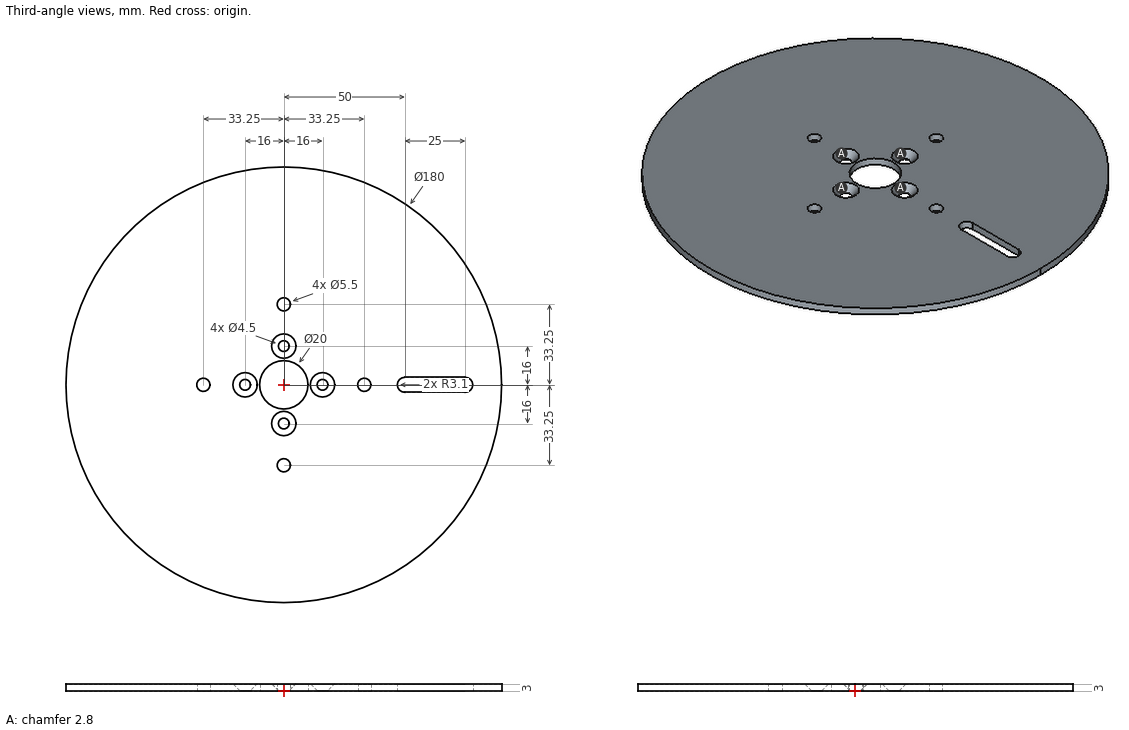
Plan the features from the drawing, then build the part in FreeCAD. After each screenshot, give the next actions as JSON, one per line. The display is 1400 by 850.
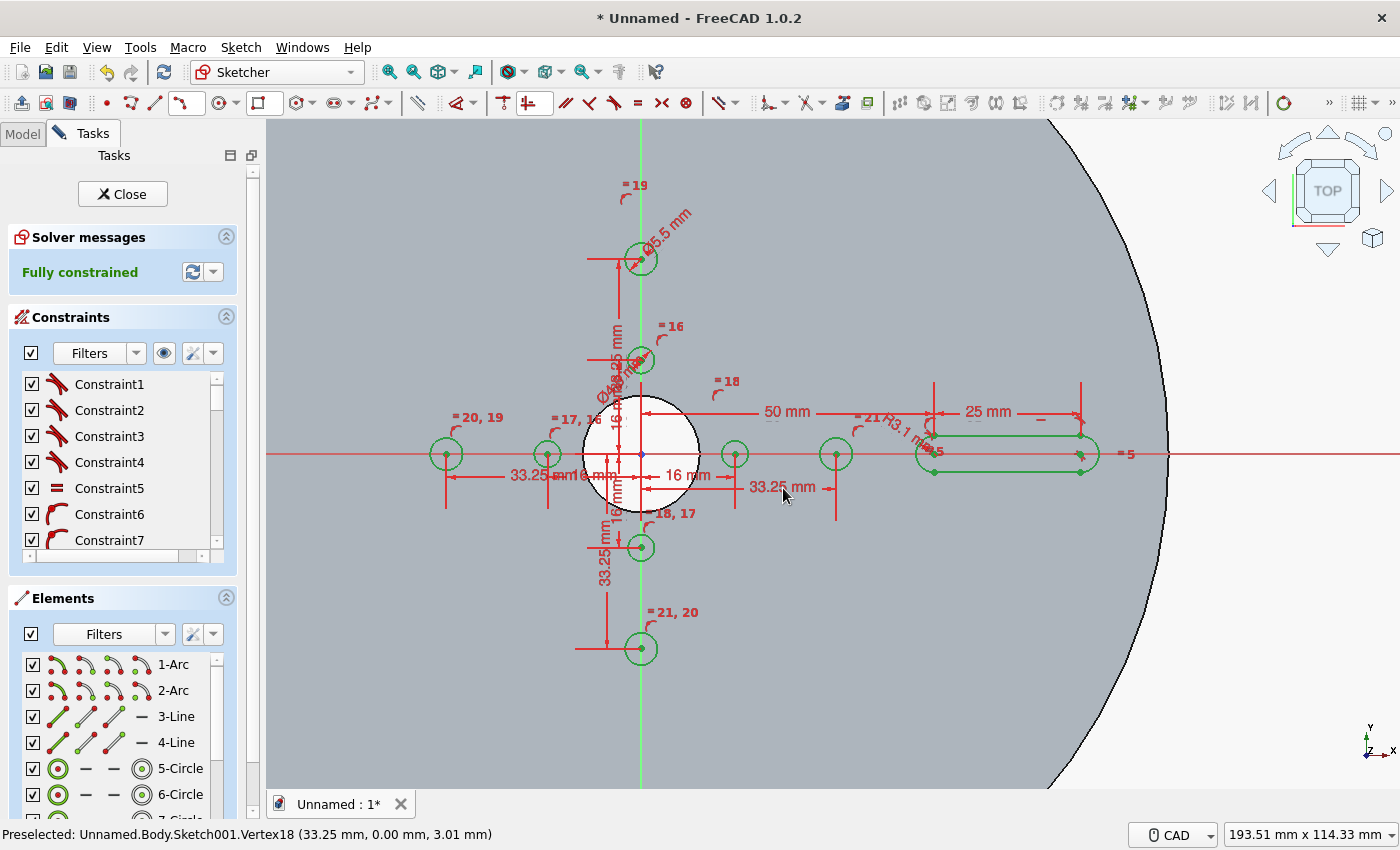
{"action": "left_click", "coordinate": [123, 194]}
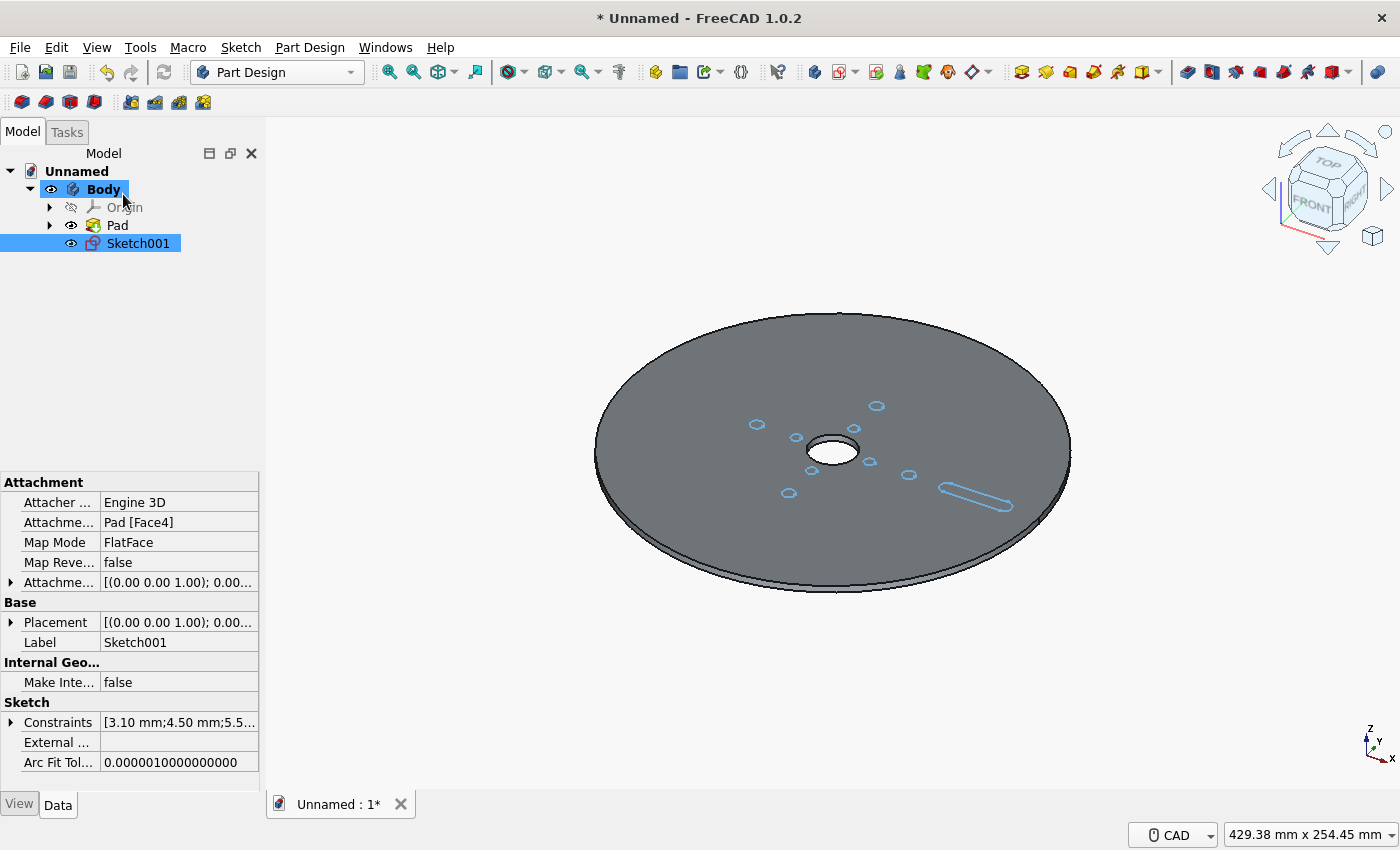
{"action": "left_click", "coordinate": [1188, 72]}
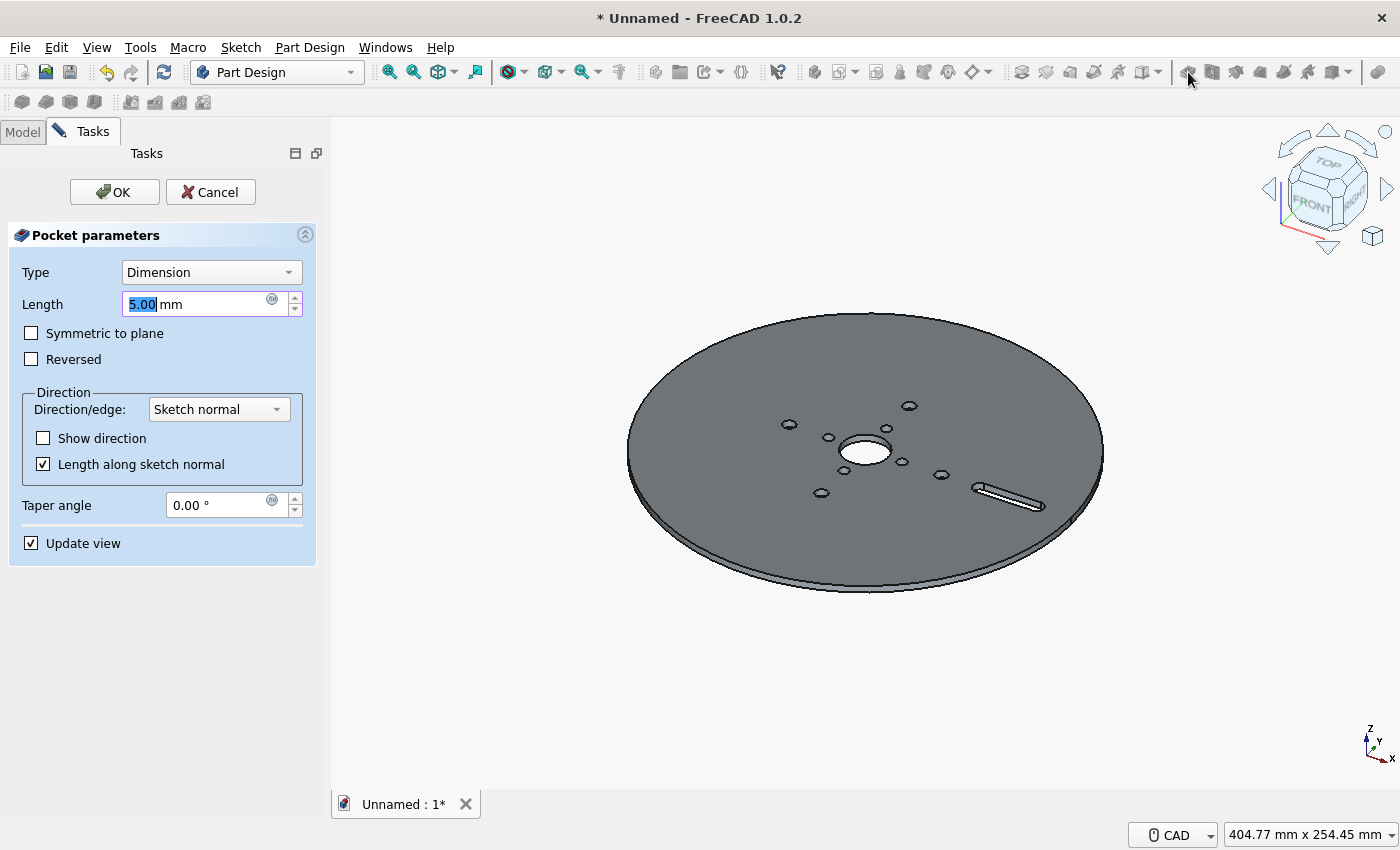
{"action": "type", "text": "3"}
{"action": "key", "text": "Tab"}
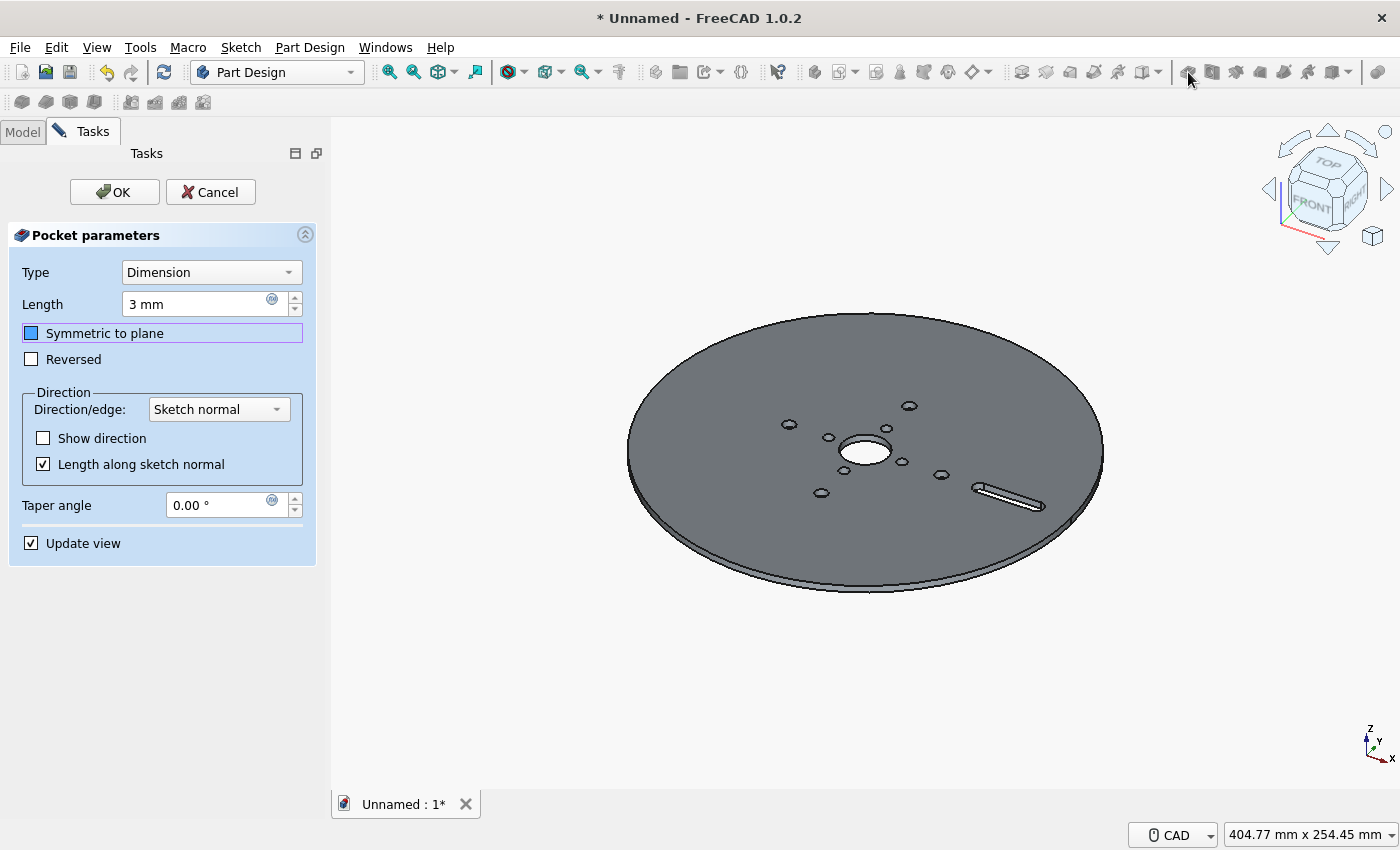
{"action": "left_click", "coordinate": [115, 192]}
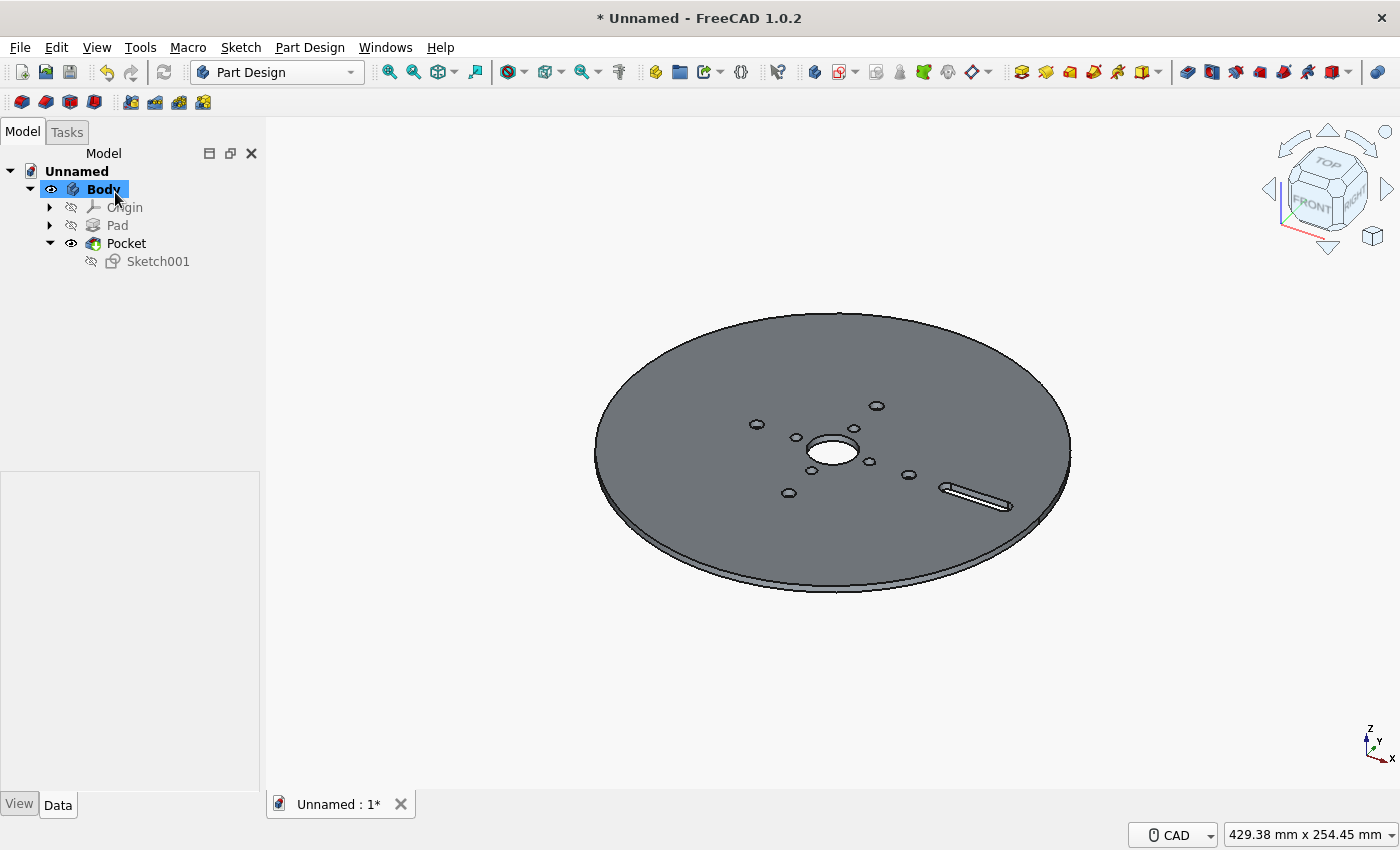
{"action": "left_click", "coordinate": [849, 426]}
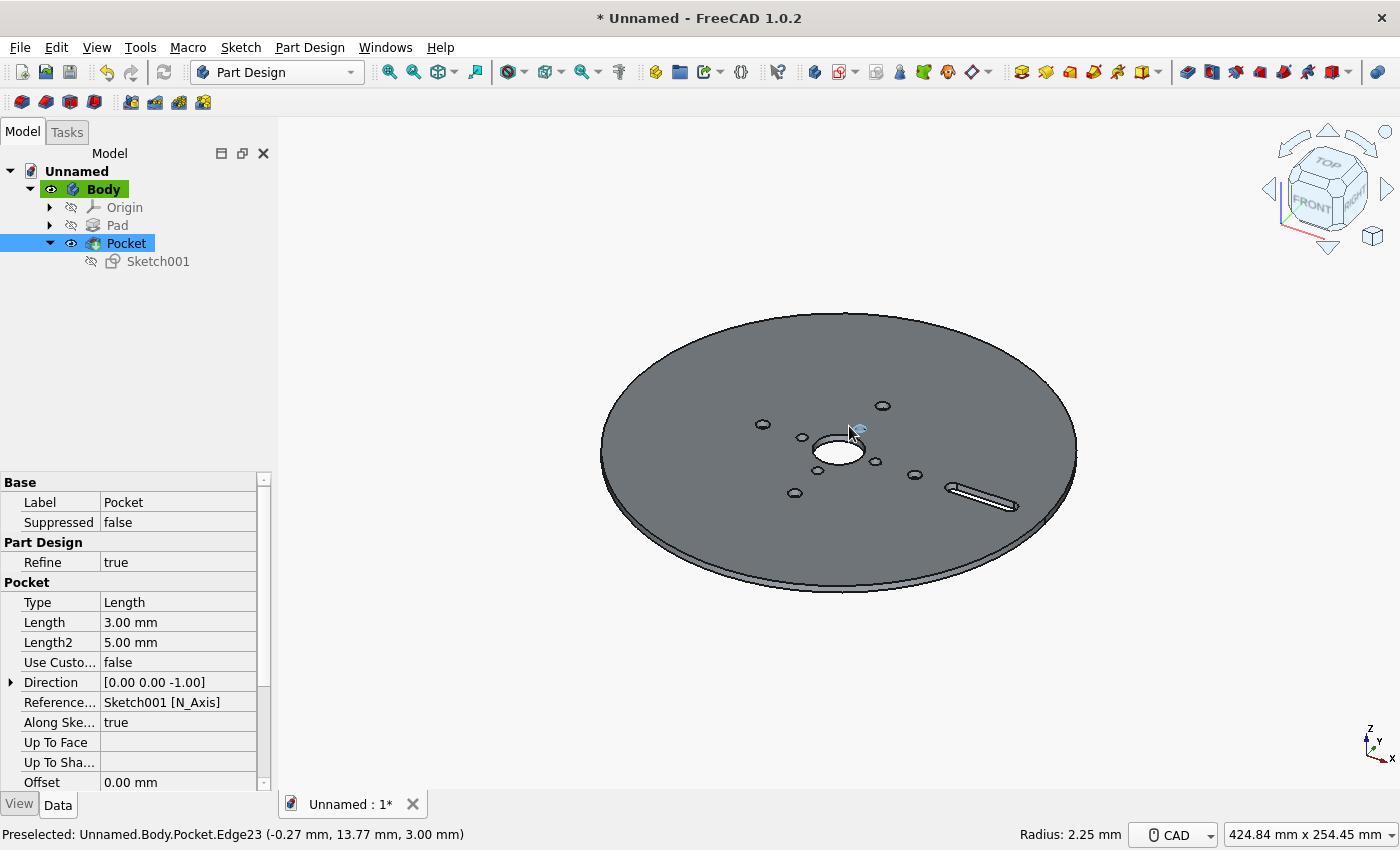
{"action": "left_click", "coordinate": [797, 435], "text": "ctrl"}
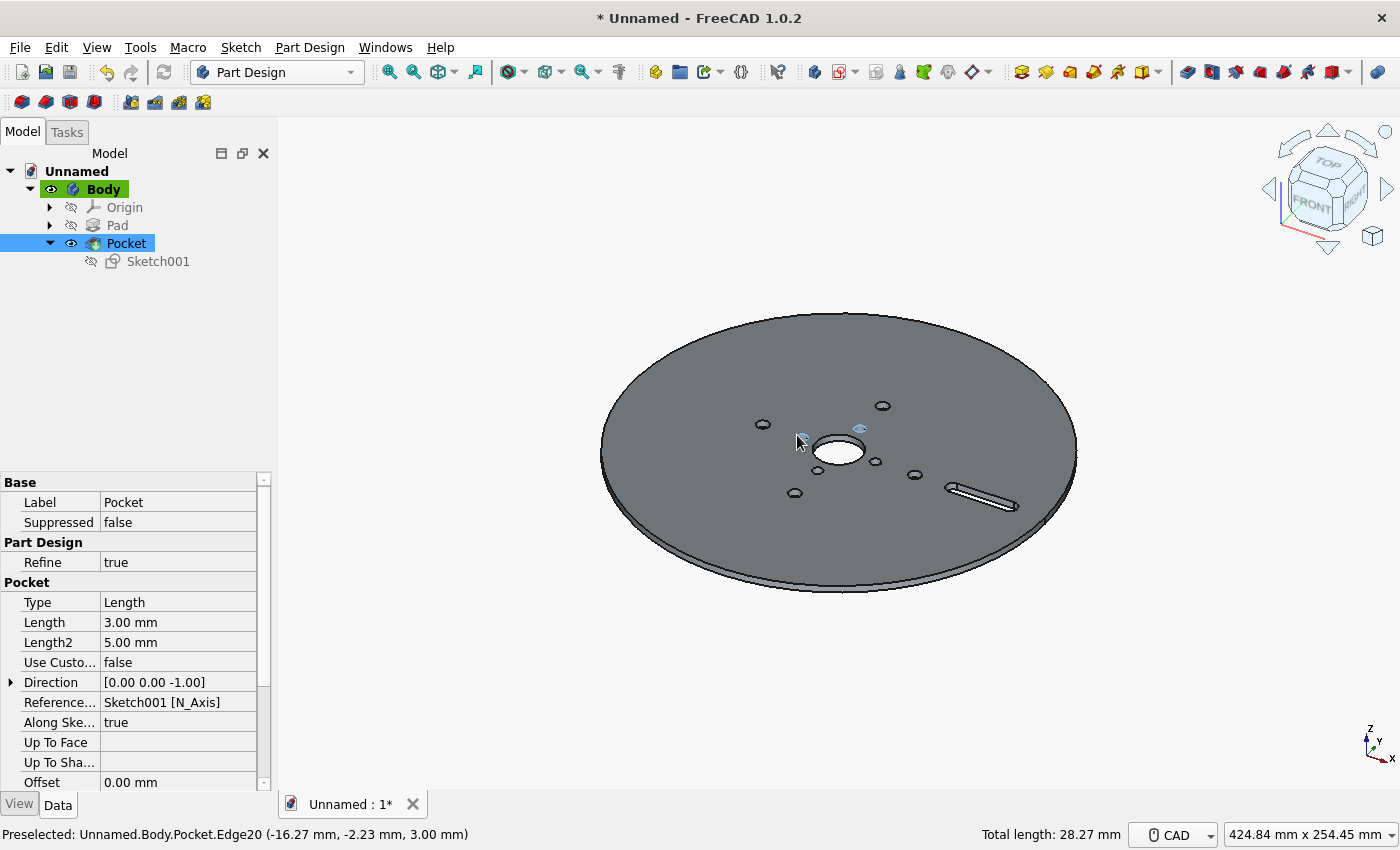
{"action": "left_click", "coordinate": [813, 468], "text": "ctrl"}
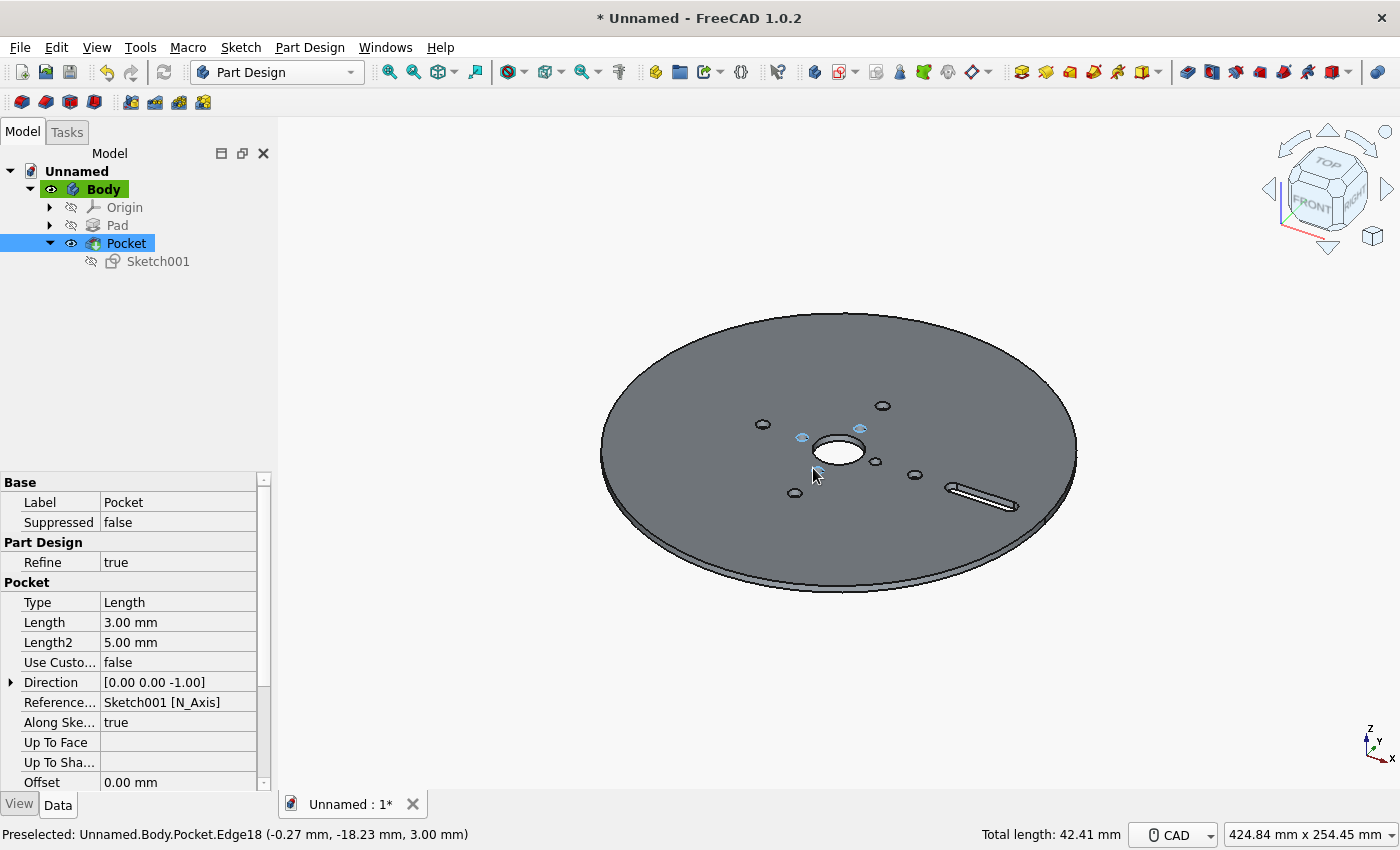
{"action": "left_click", "coordinate": [870, 459], "text": "ctrl"}